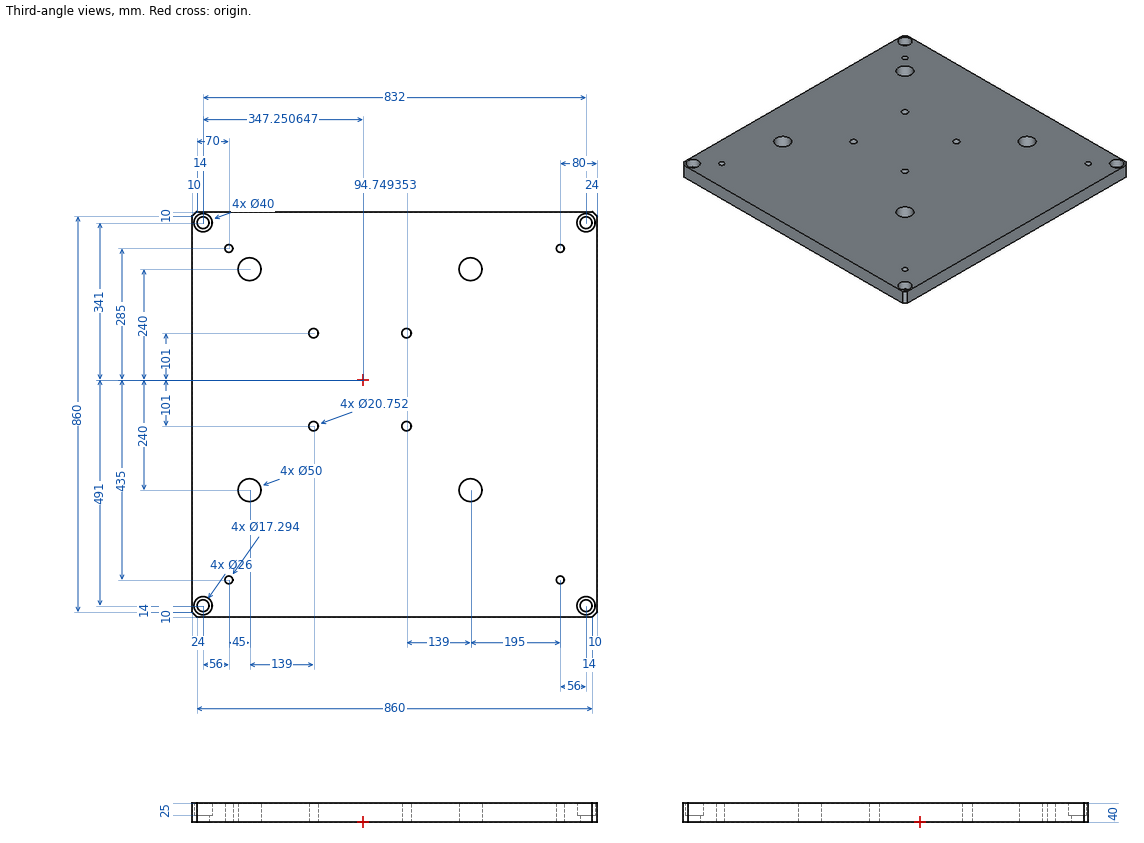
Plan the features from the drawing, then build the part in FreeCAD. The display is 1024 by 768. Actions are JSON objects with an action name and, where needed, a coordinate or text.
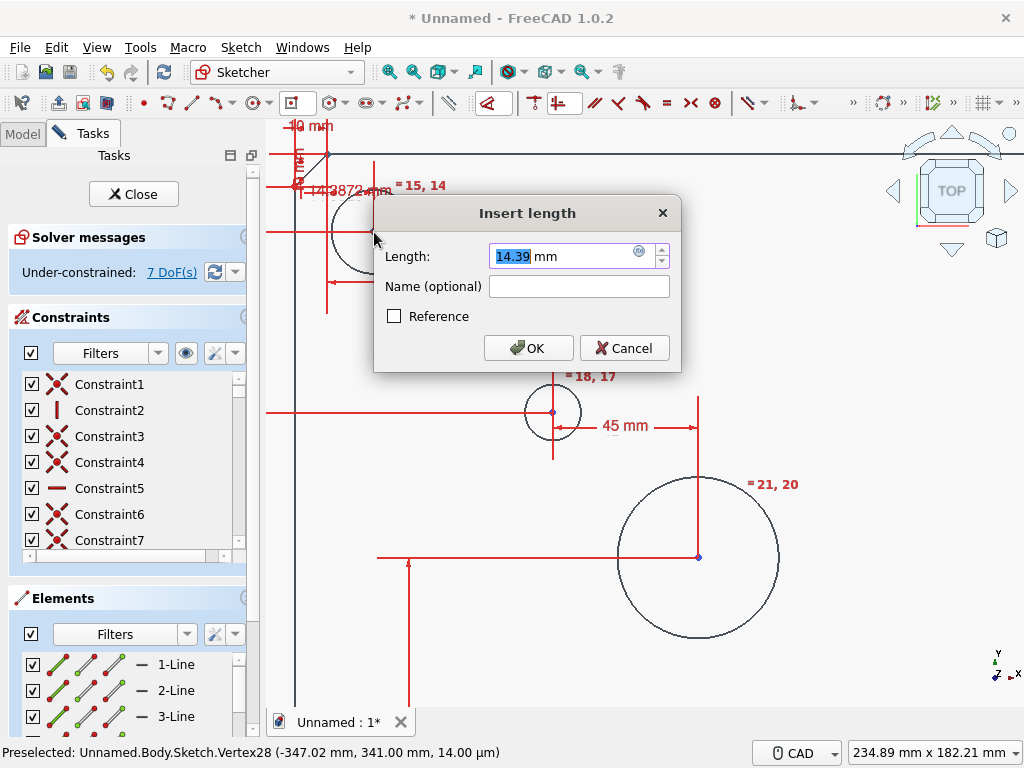
{"action": "type", "text": "14"}
{"action": "key", "text": "Return"}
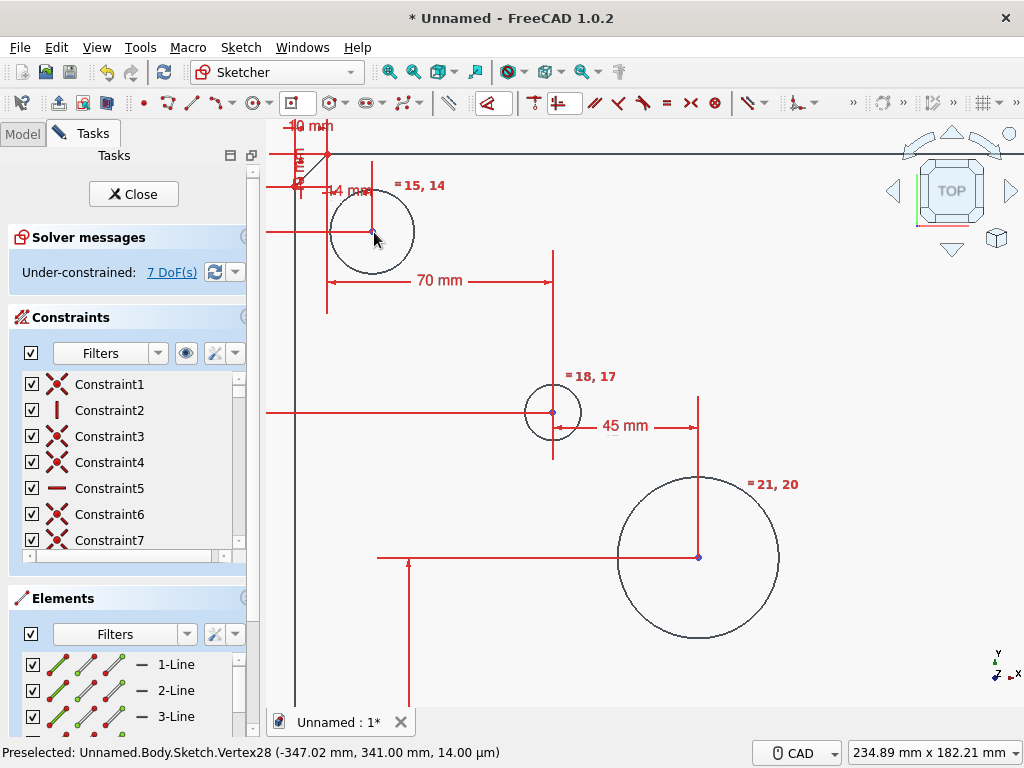
{"action": "scroll", "coordinate": [398, 231], "scroll_direction": "down", "scroll_amount": 10}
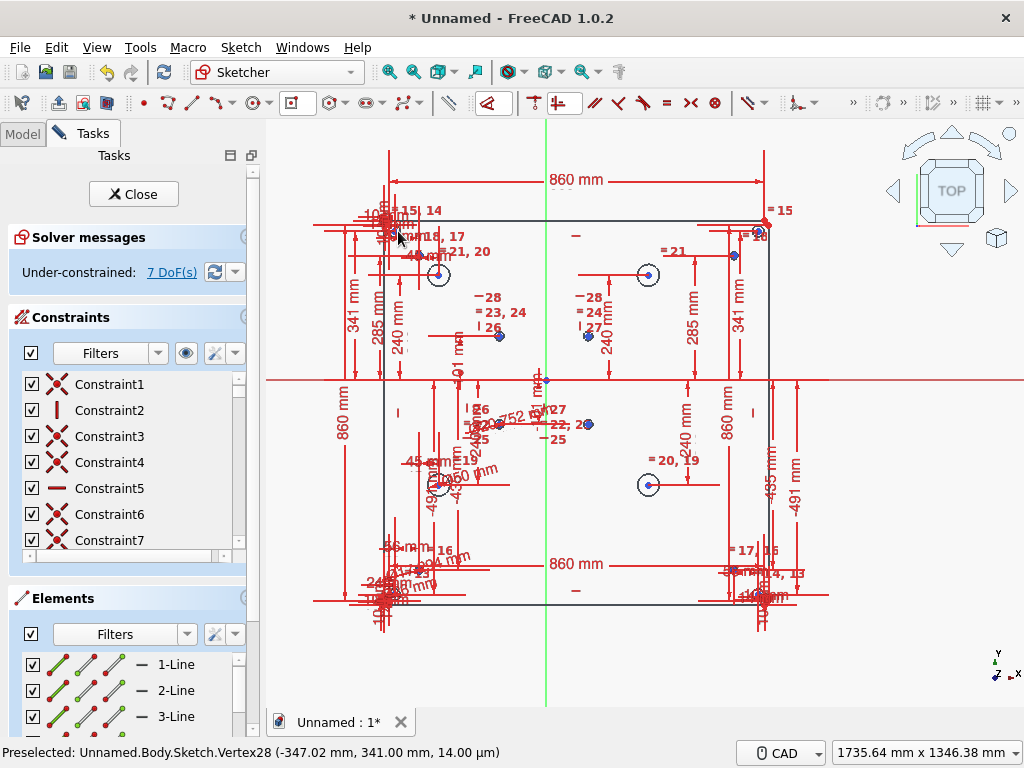
{"action": "scroll", "coordinate": [769, 225], "scroll_direction": "up", "scroll_amount": 4}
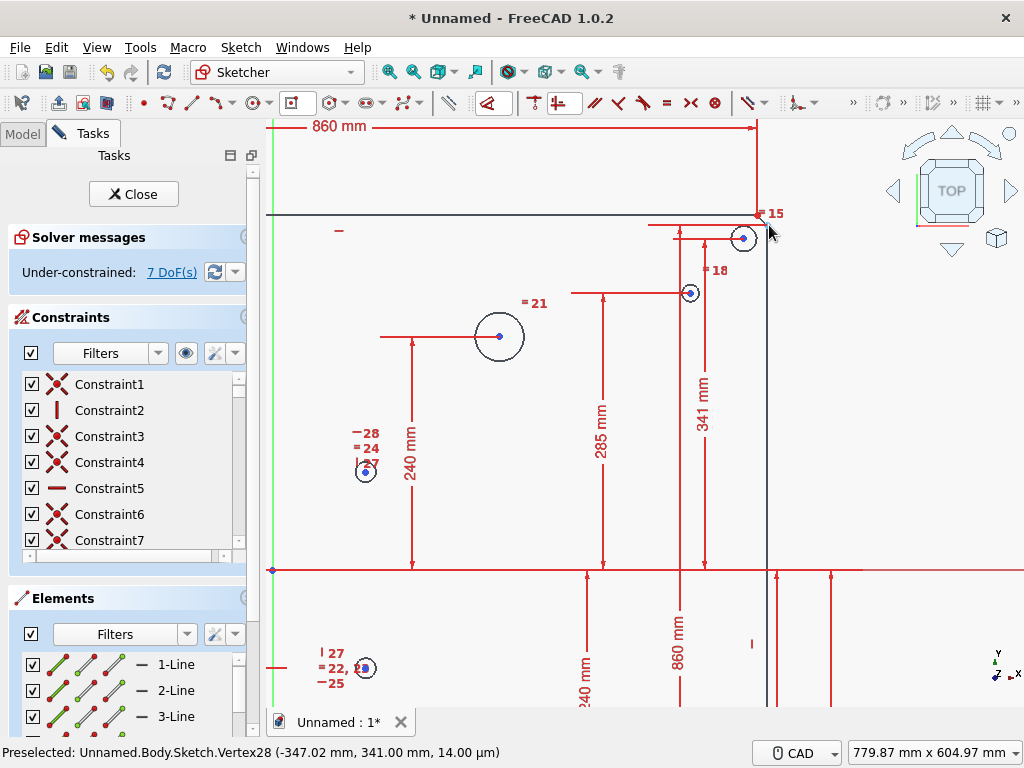
{"action": "left_click", "coordinate": [767, 225]}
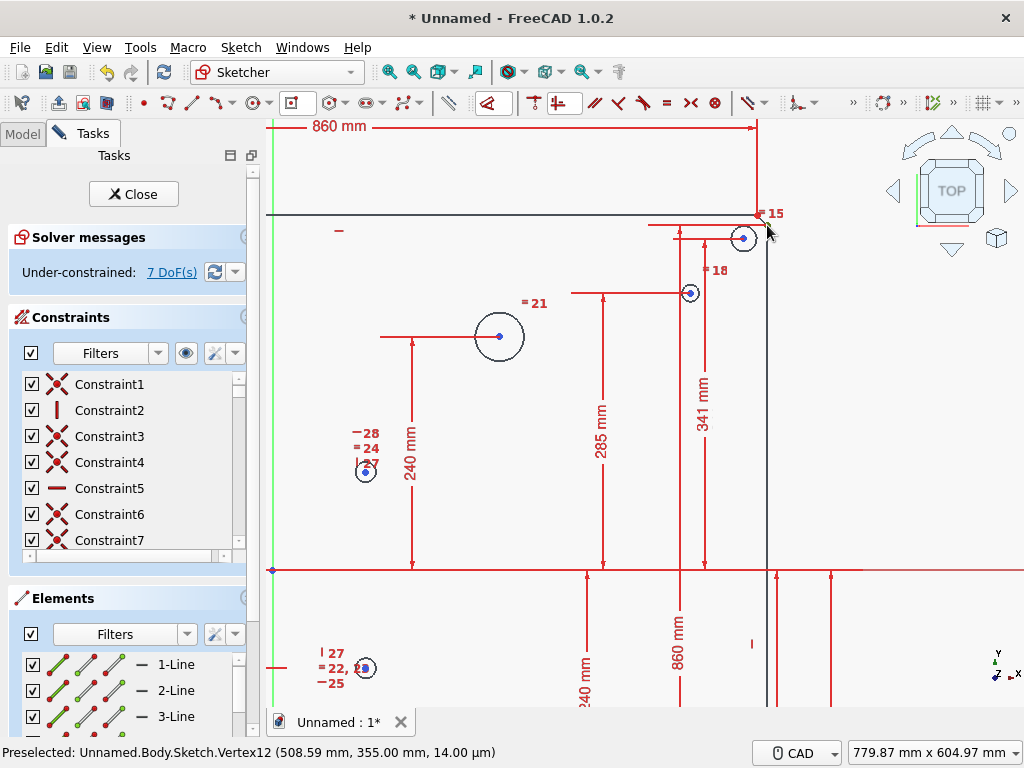
{"action": "left_click", "coordinate": [691, 293]}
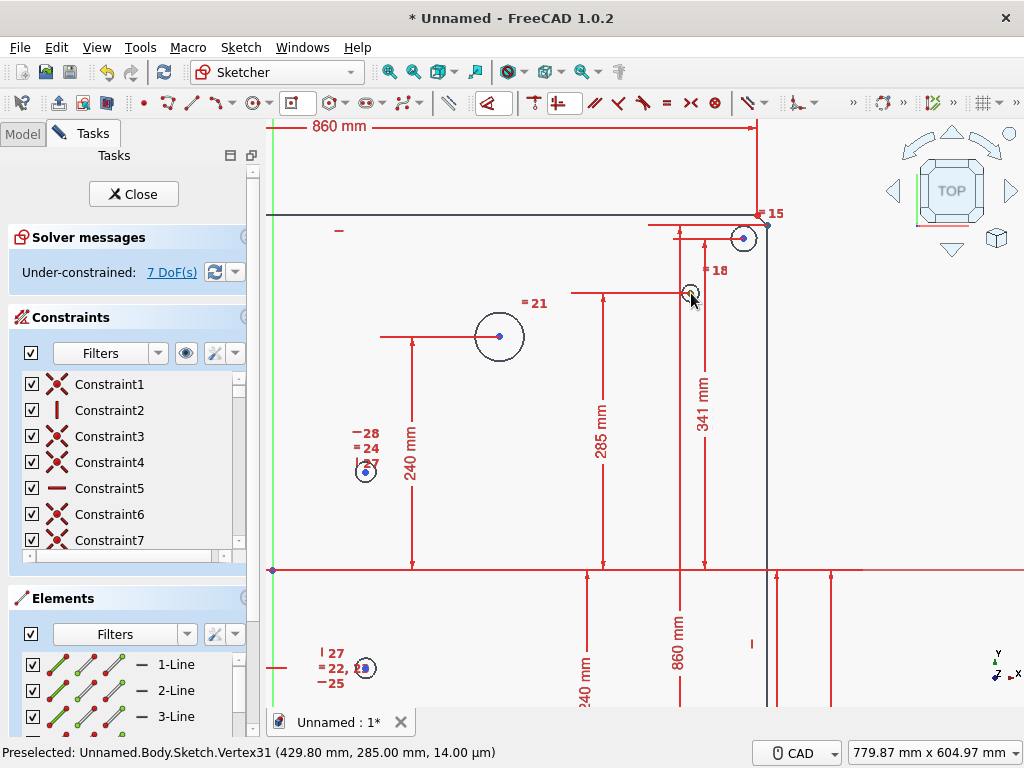
{"action": "key", "text": "l"}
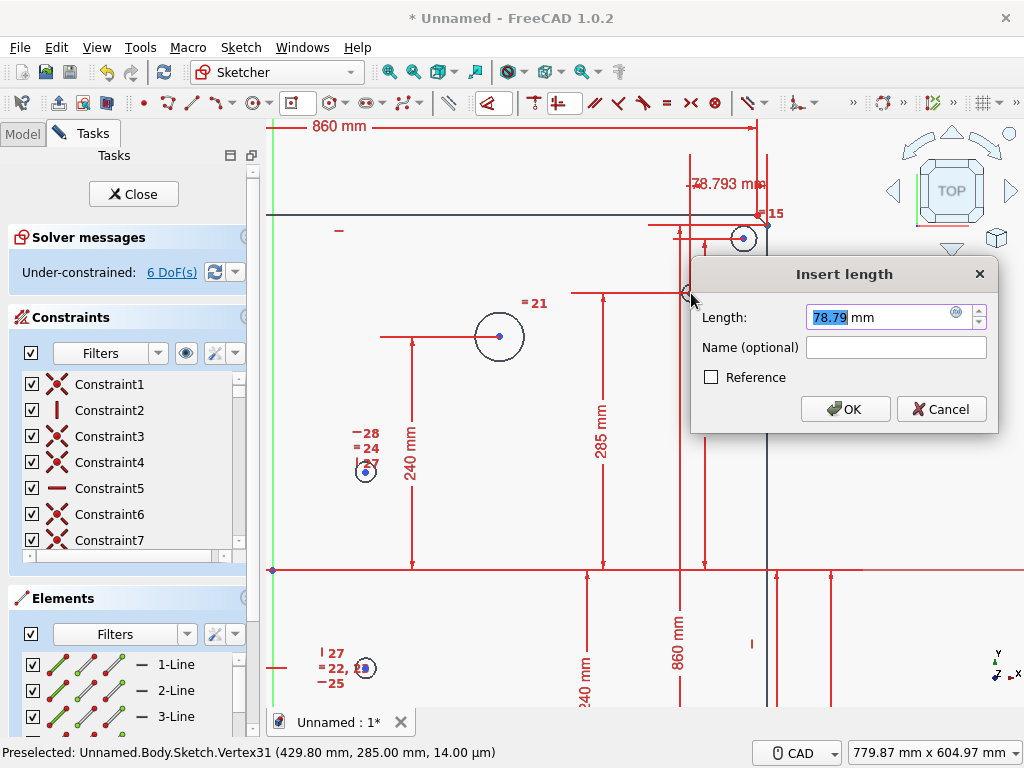
{"action": "type", "text": "80"}
{"action": "key", "text": "Return"}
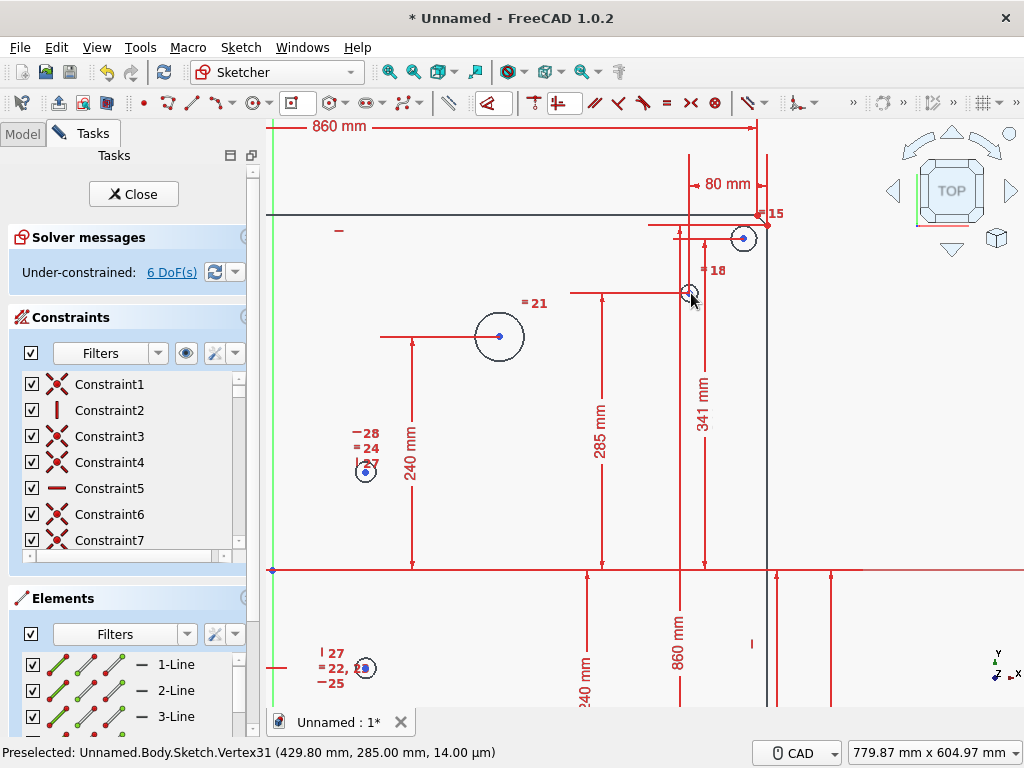
{"action": "scroll", "coordinate": [767, 225], "scroll_direction": "up", "scroll_amount": 3}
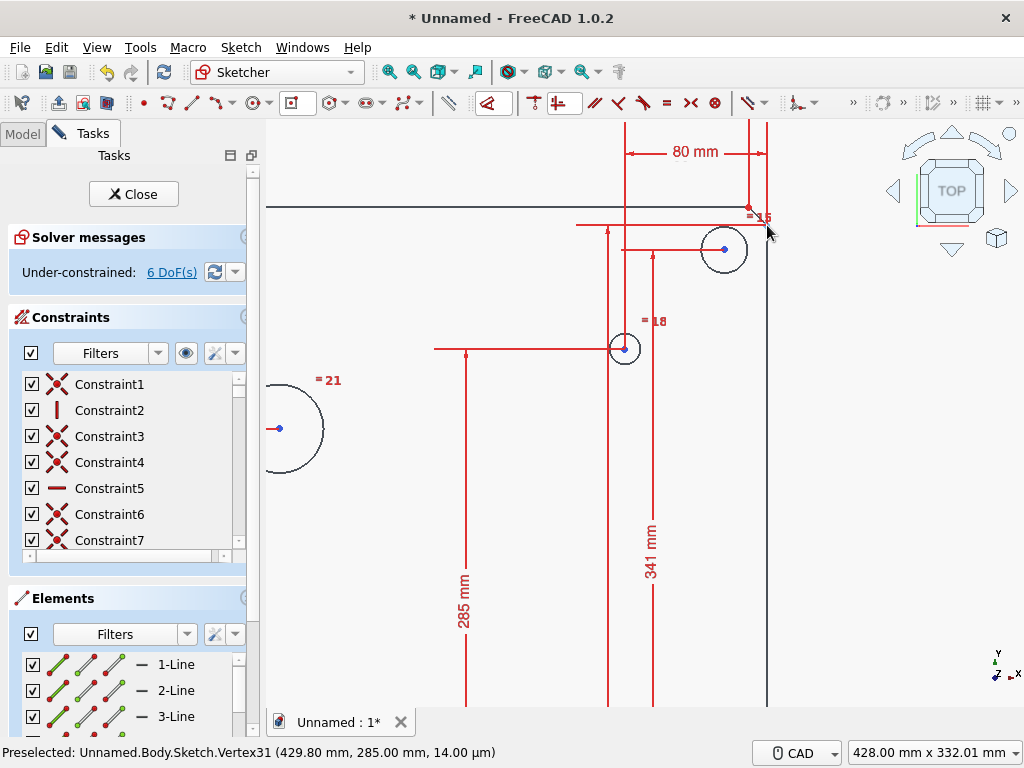
{"action": "left_click", "coordinate": [767, 225]}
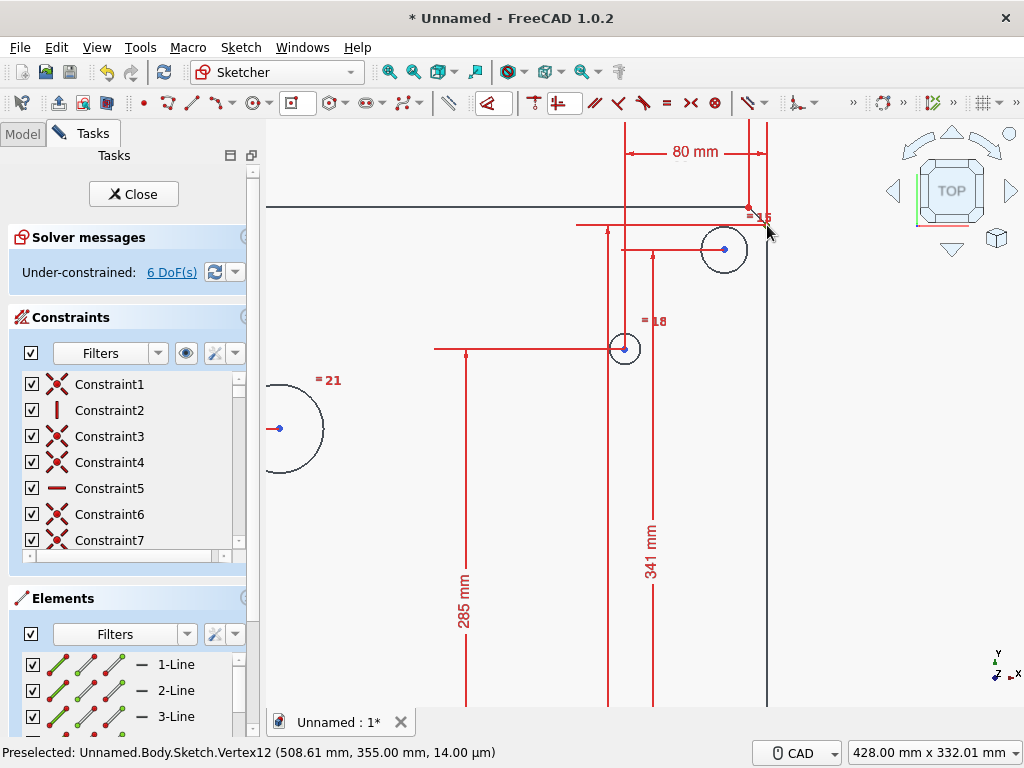
{"action": "left_click", "coordinate": [724, 250]}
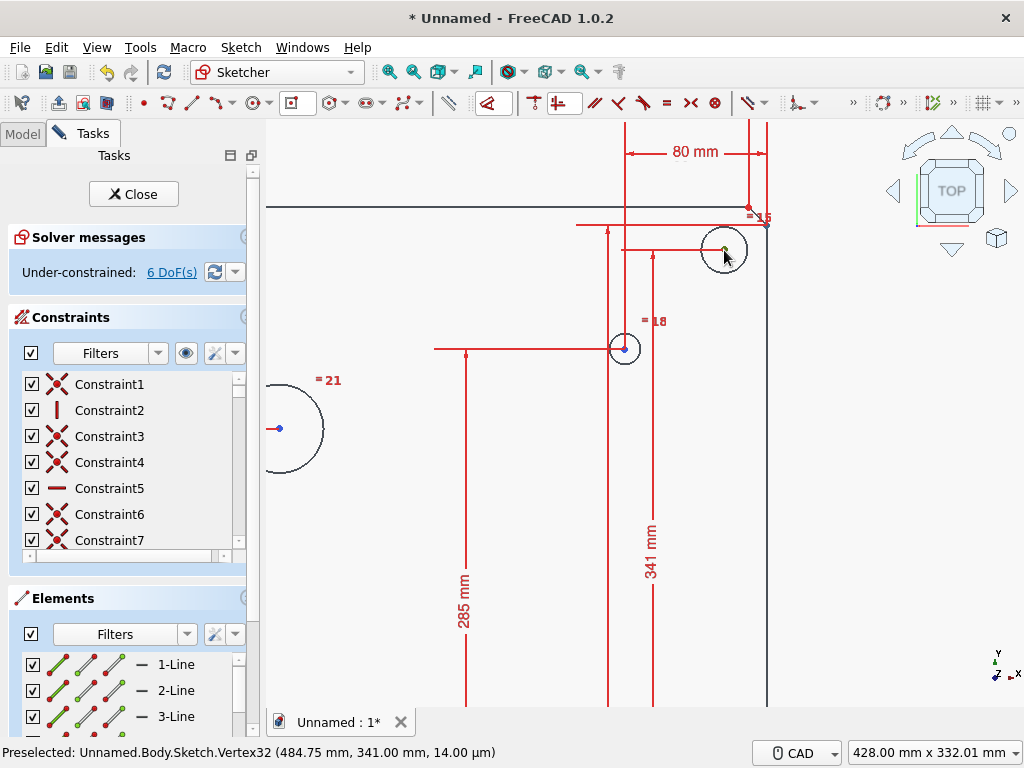
{"action": "key", "text": "l"}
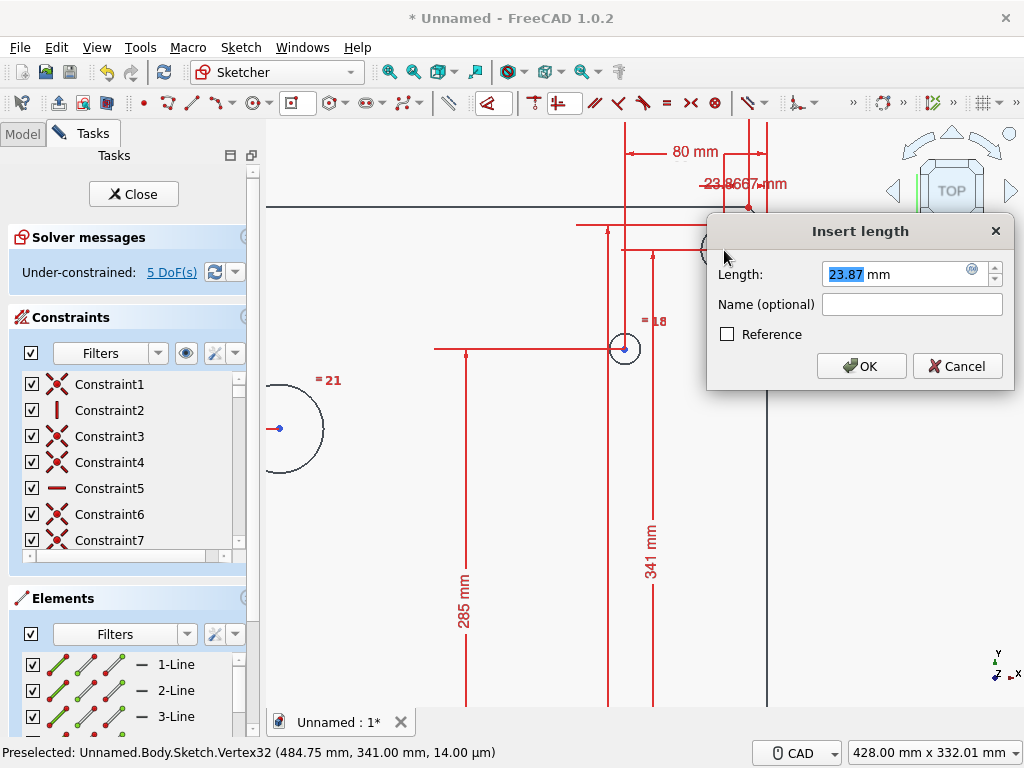
{"action": "type", "text": "24"}
{"action": "key", "text": "Return"}